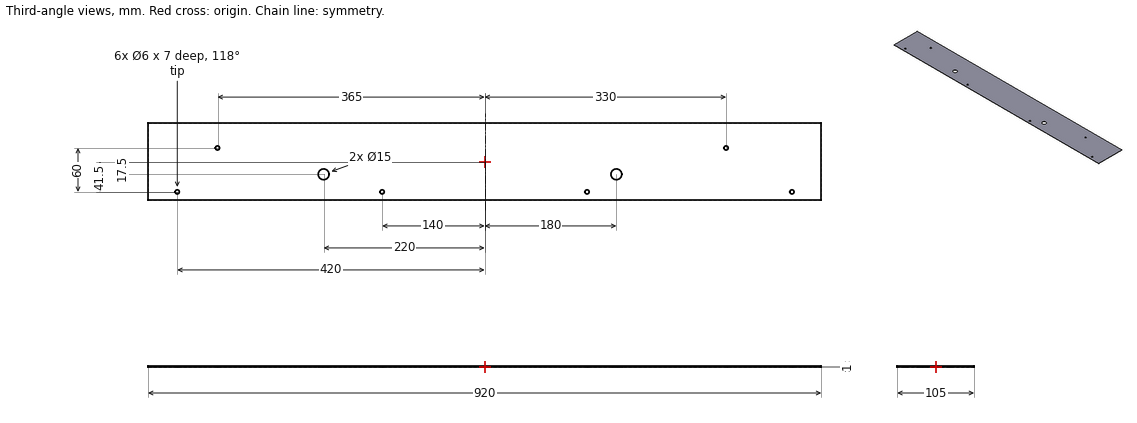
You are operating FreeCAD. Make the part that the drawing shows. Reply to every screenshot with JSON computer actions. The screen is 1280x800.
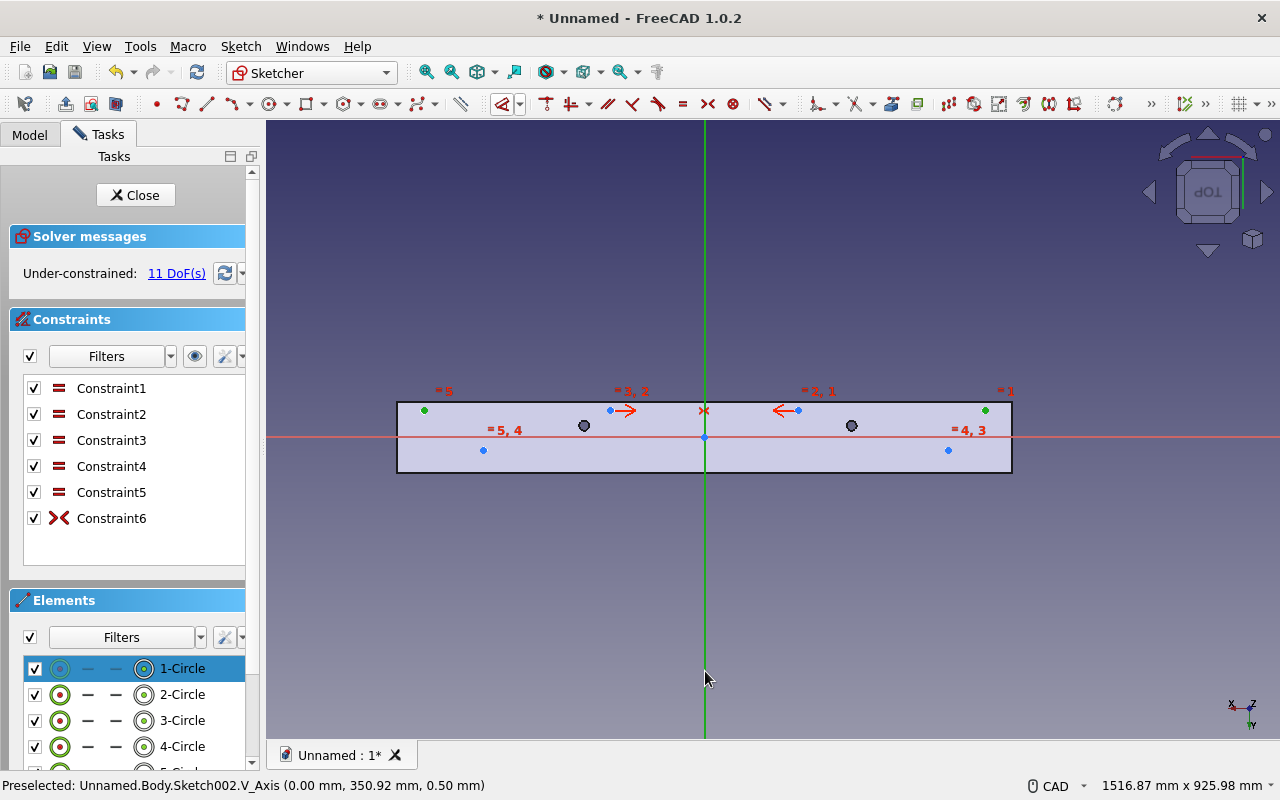
{"action": "left_click", "coordinate": [708, 104]}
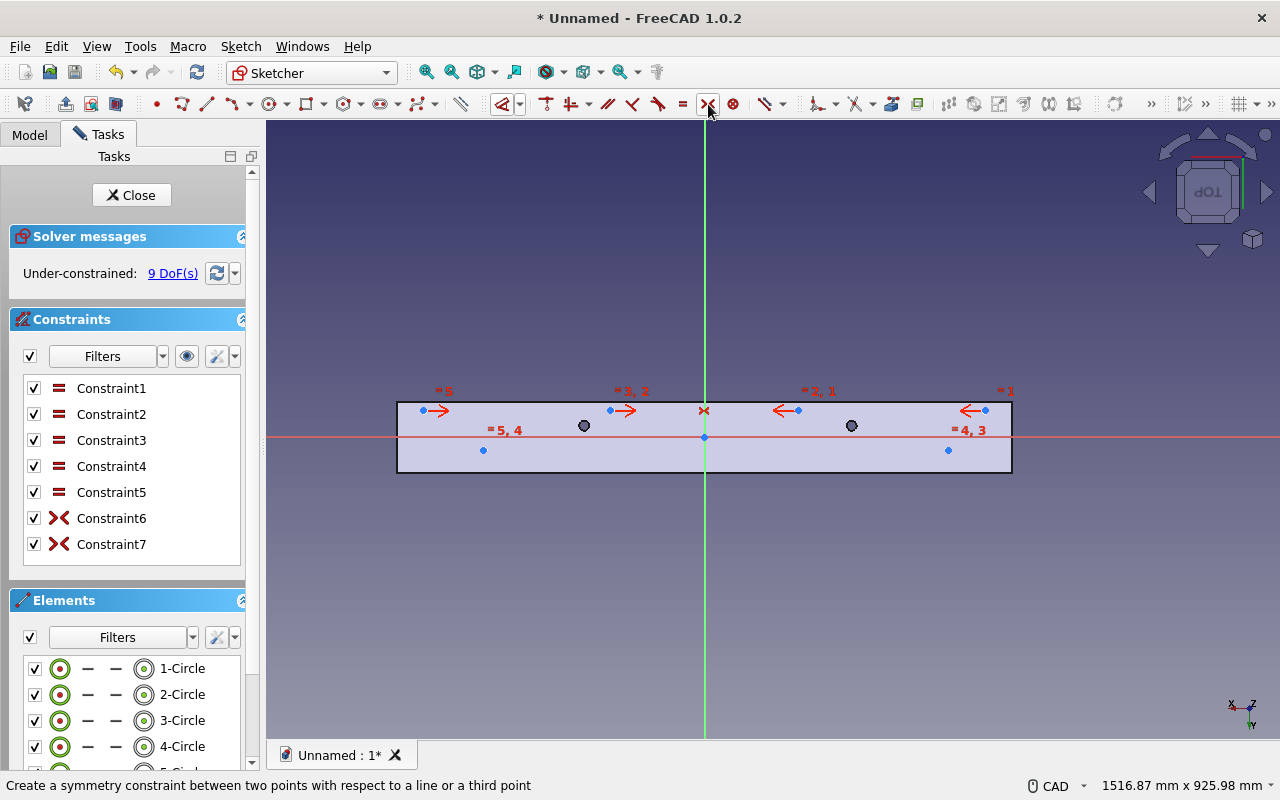
{"action": "scroll", "coordinate": [982, 411], "scroll_direction": "up", "scroll_amount": 12}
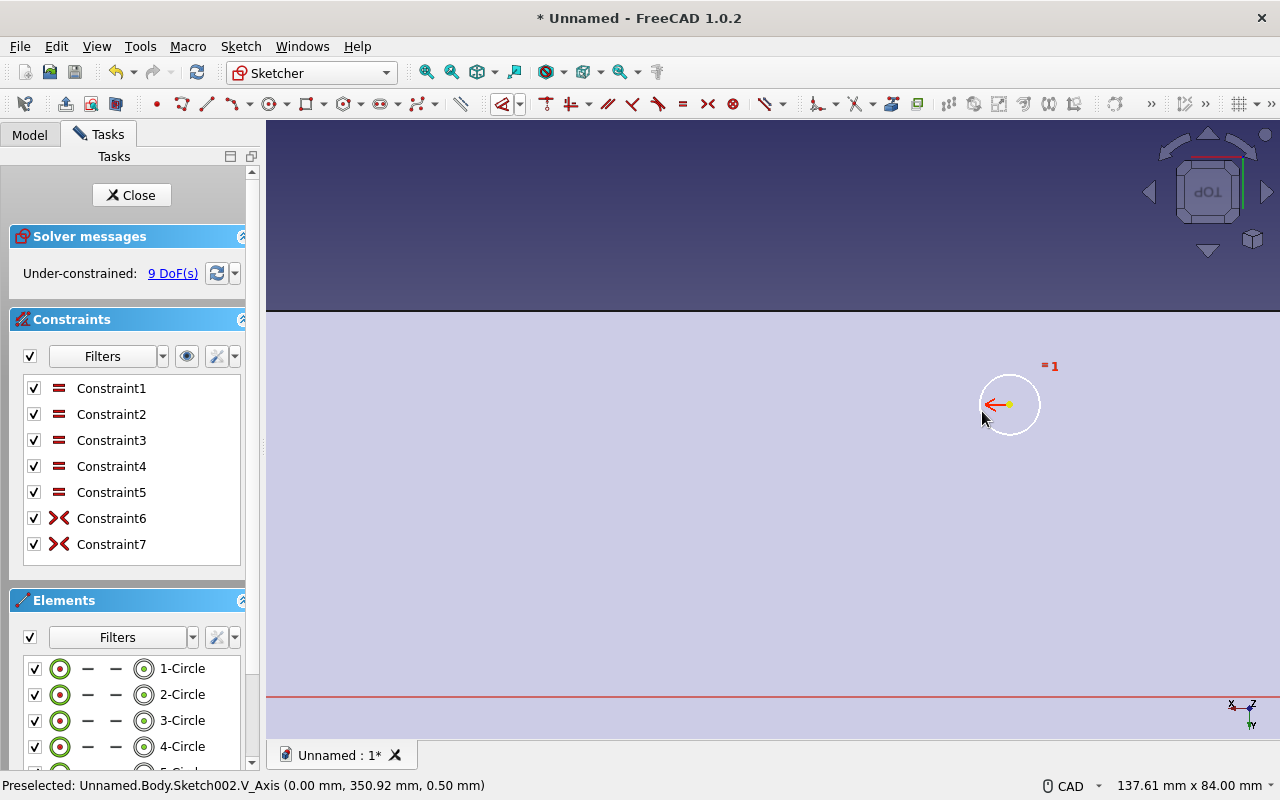
{"action": "left_click", "coordinate": [1040, 406]}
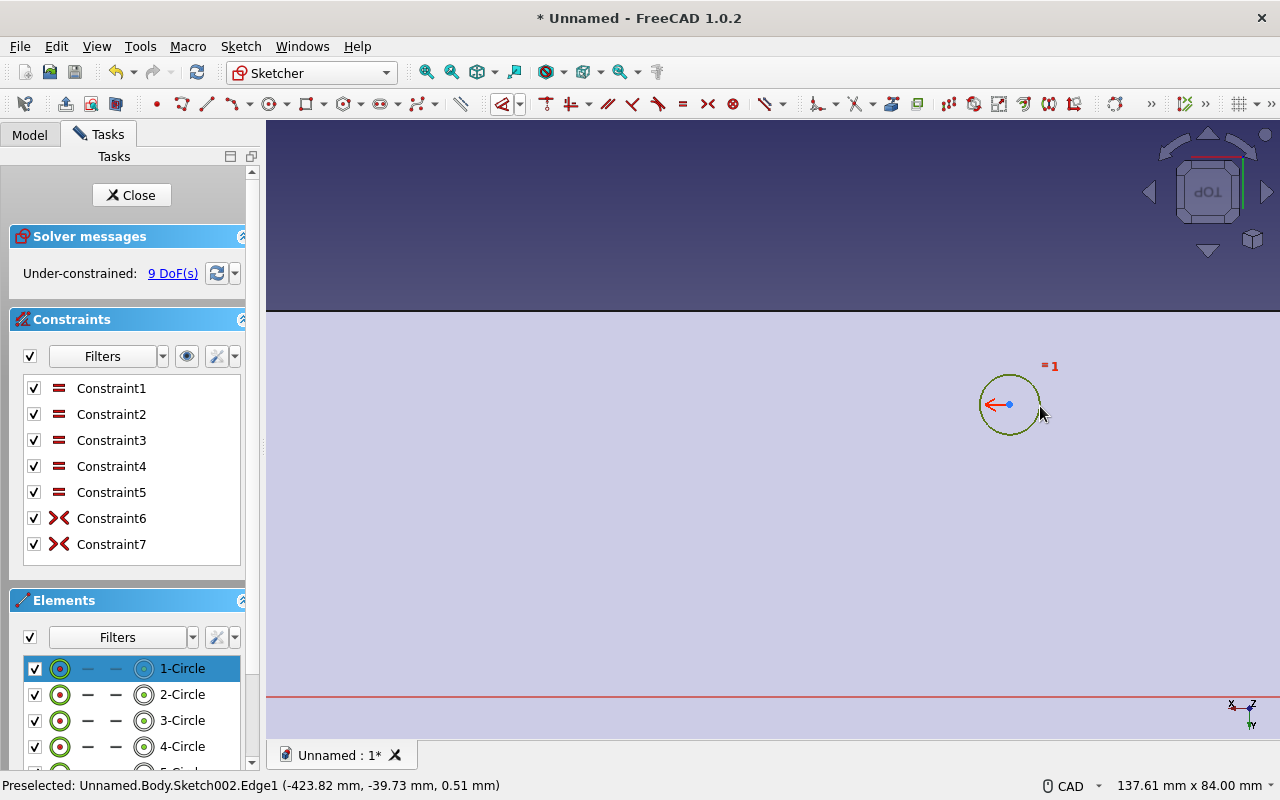
{"action": "left_click", "coordinate": [520, 104]}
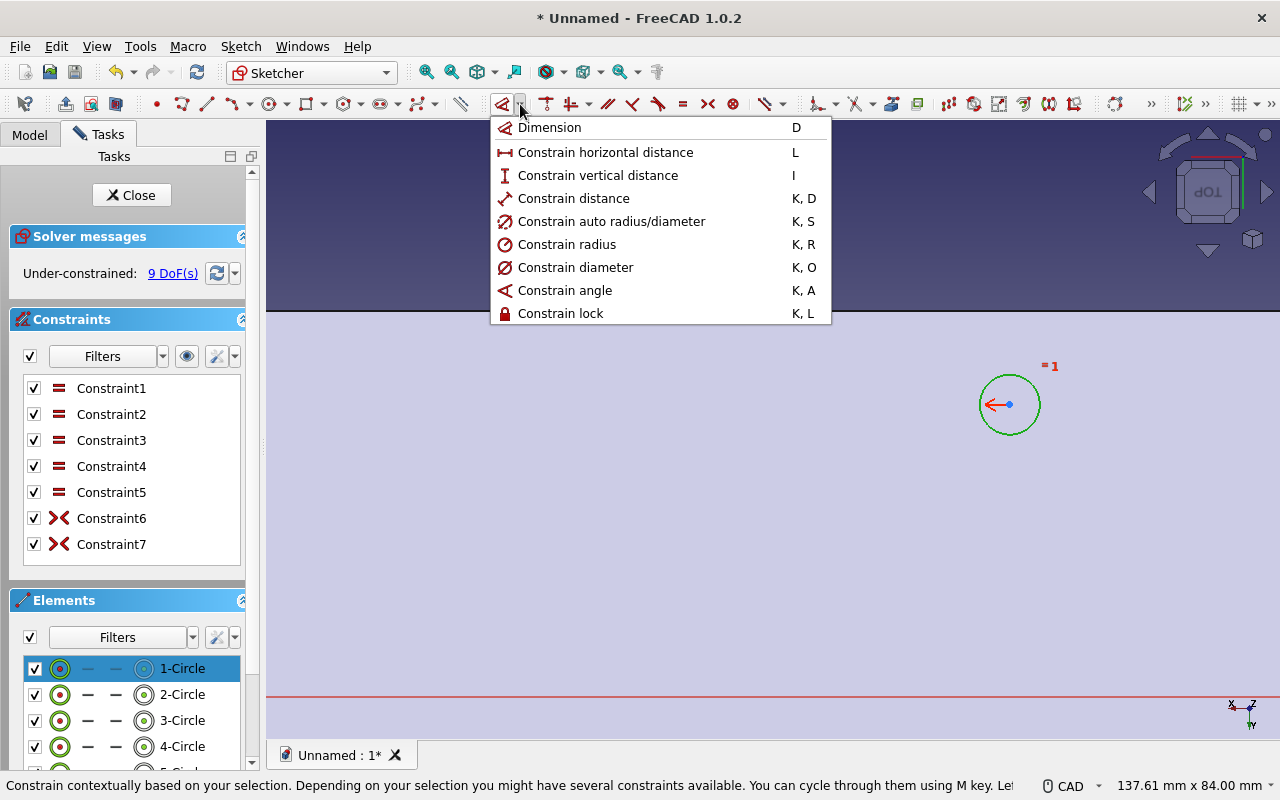
{"action": "left_click", "coordinate": [661, 268]}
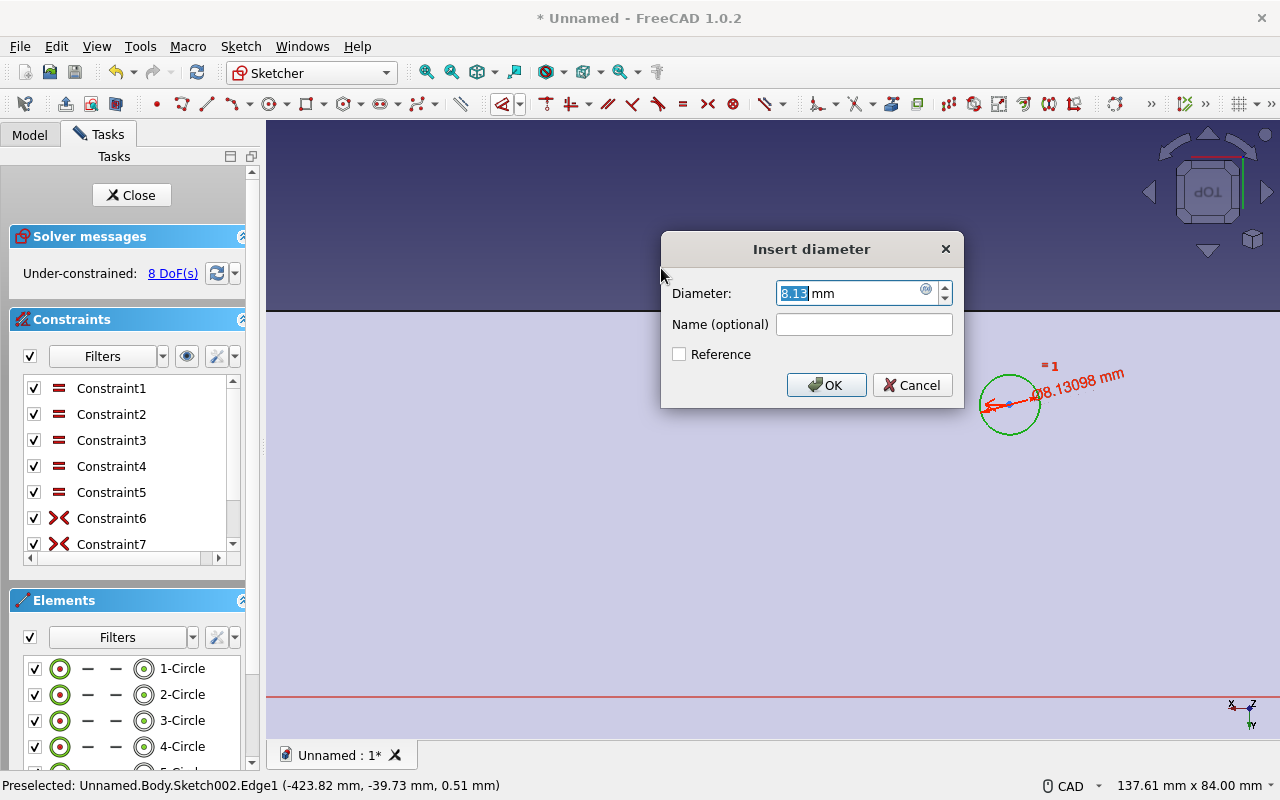
{"action": "type", "text": "6"}
{"action": "key", "text": "Return"}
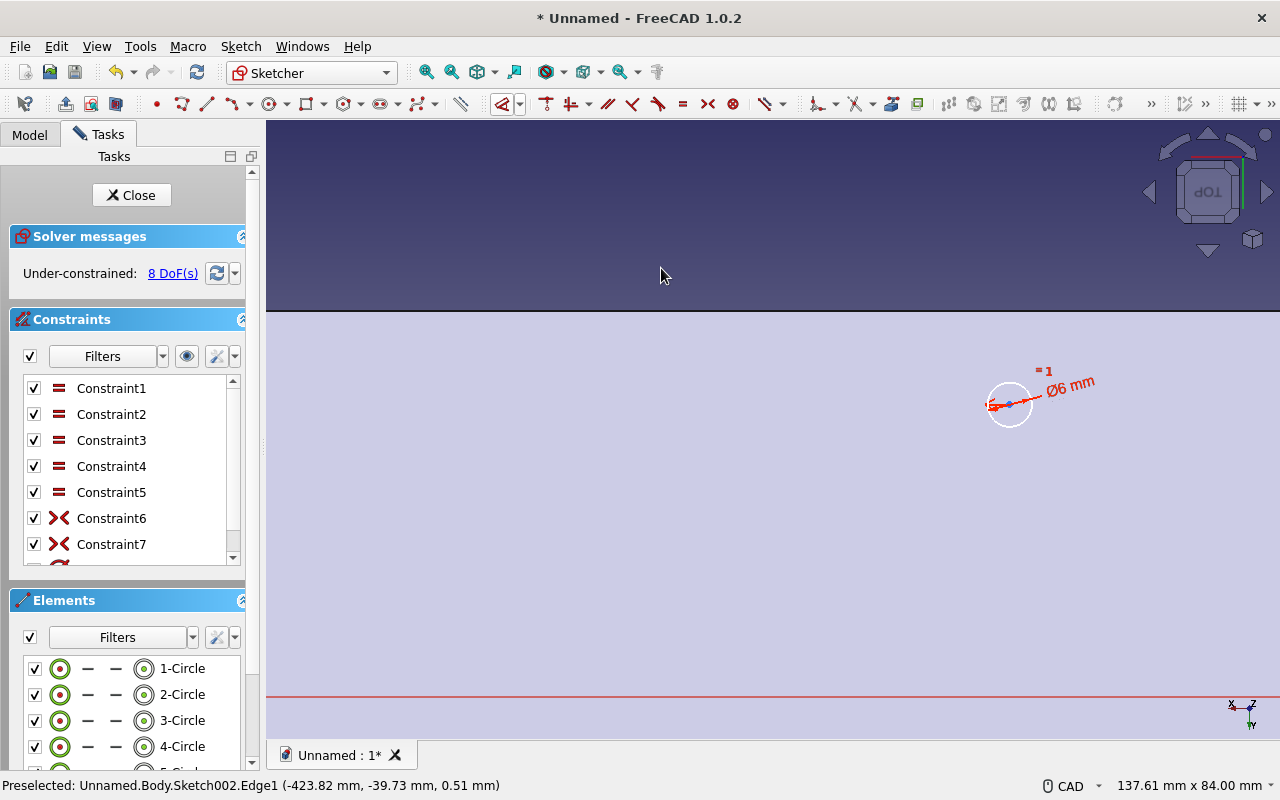
{"action": "scroll", "coordinate": [983, 411], "scroll_direction": "down", "scroll_amount": 12}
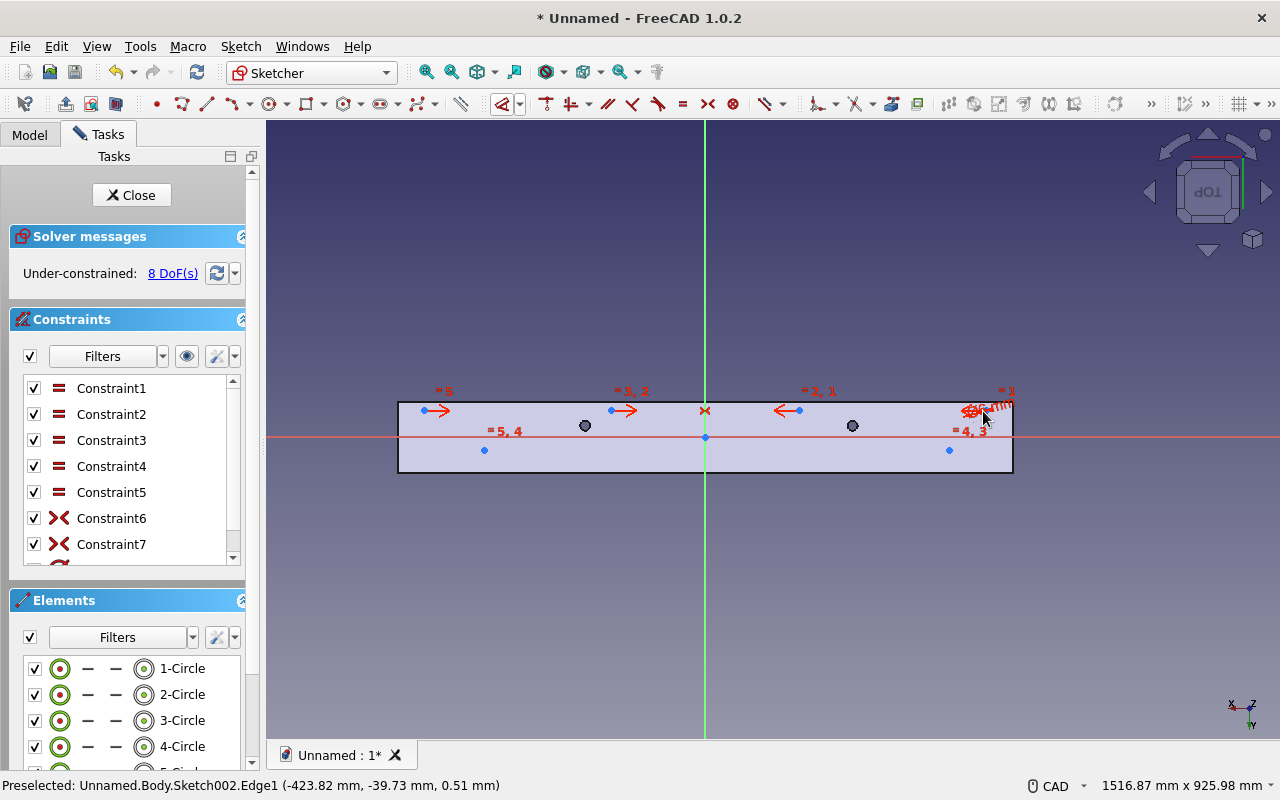
{"action": "left_click", "coordinate": [986, 411]}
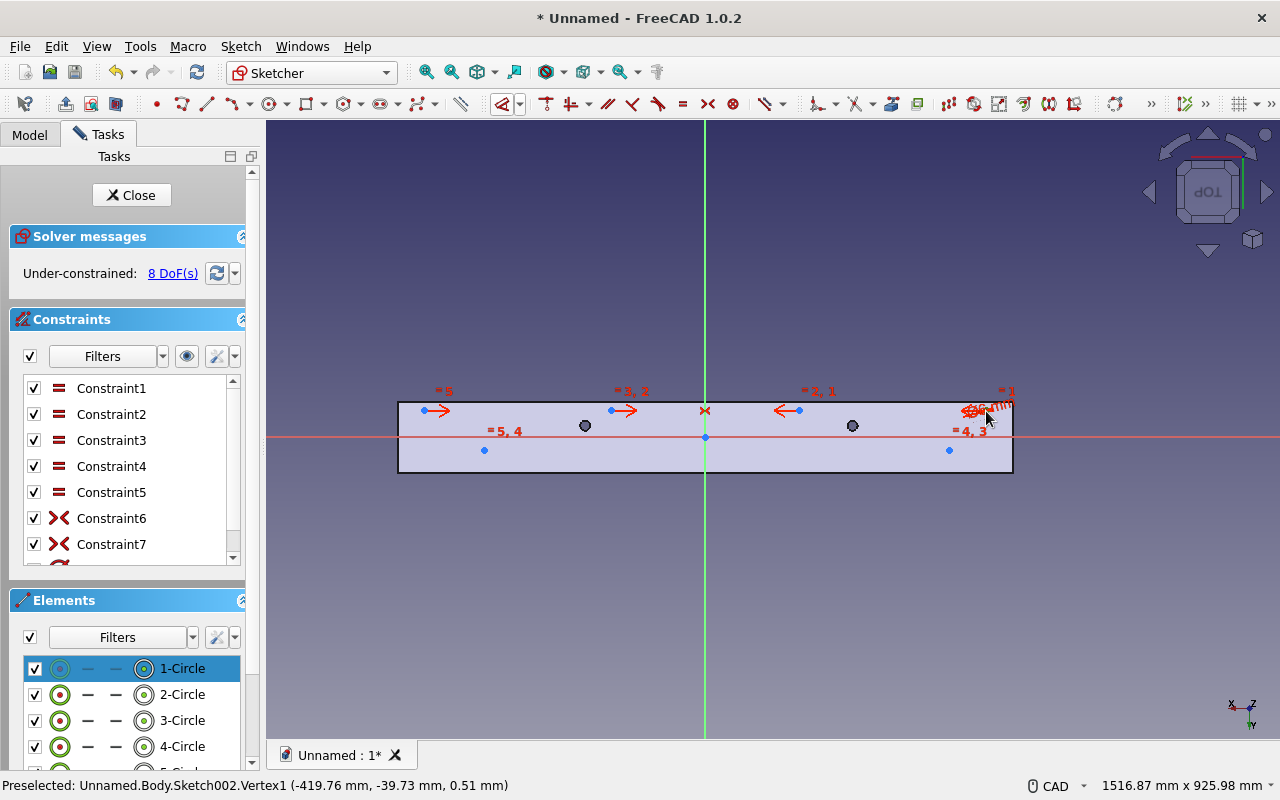
{"action": "left_click", "coordinate": [520, 104]}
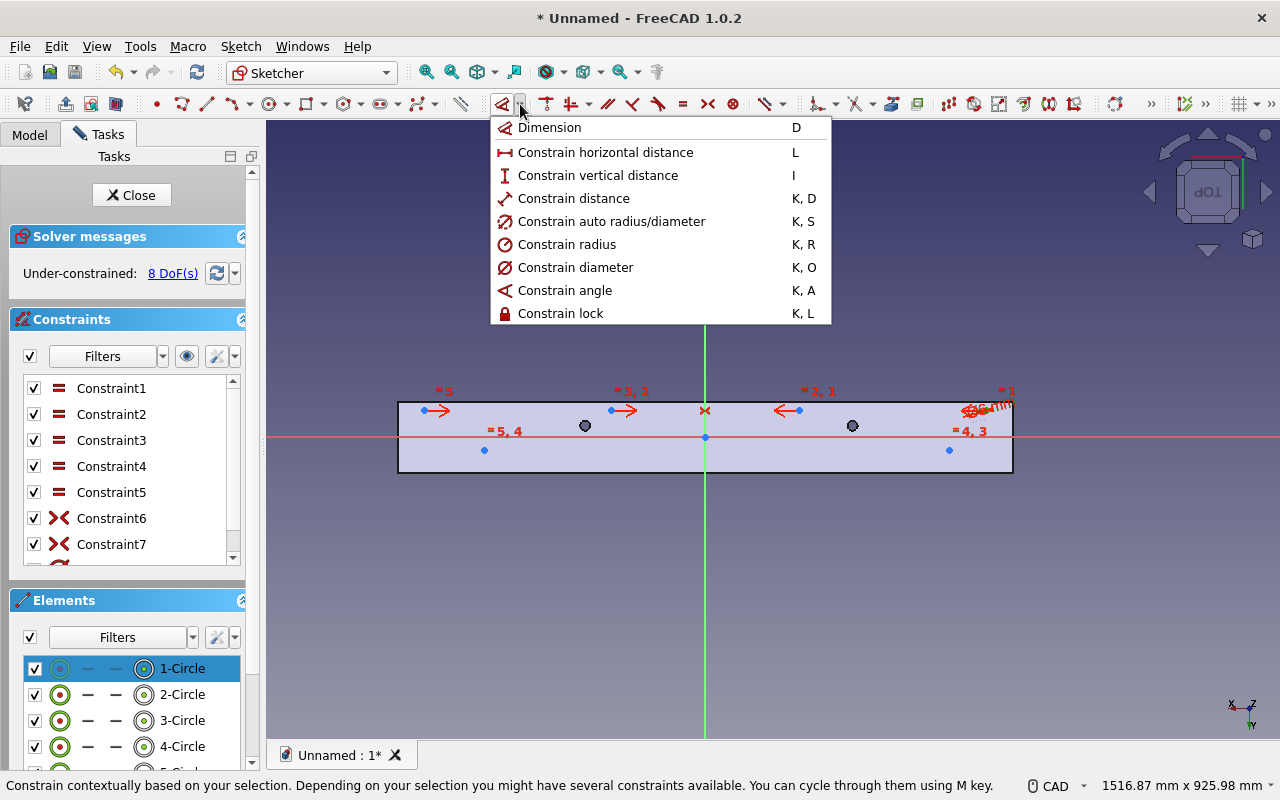
{"action": "left_click", "coordinate": [661, 152]}